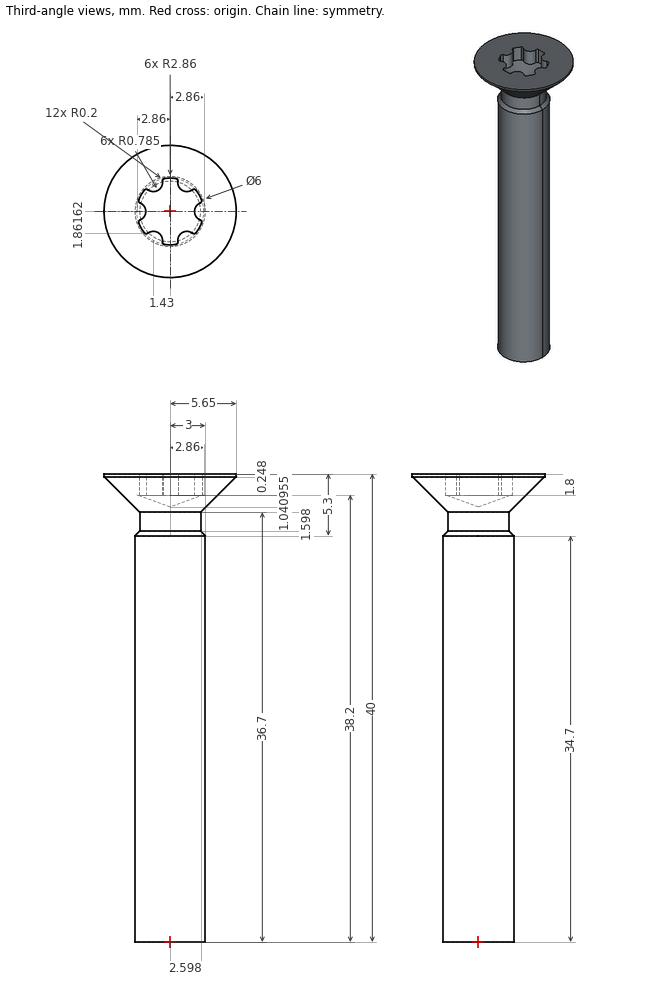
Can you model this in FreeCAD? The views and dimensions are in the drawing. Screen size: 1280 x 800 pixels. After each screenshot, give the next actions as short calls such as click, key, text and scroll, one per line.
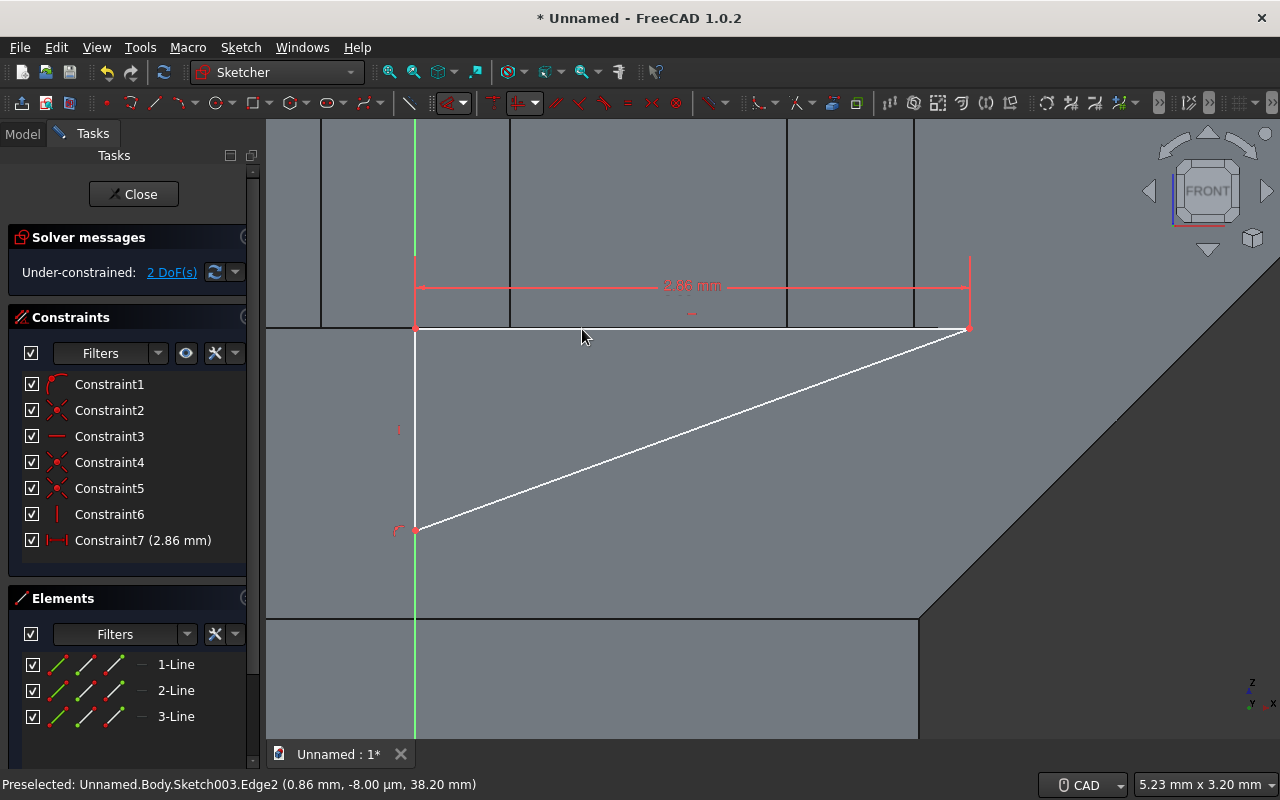
click(415, 329)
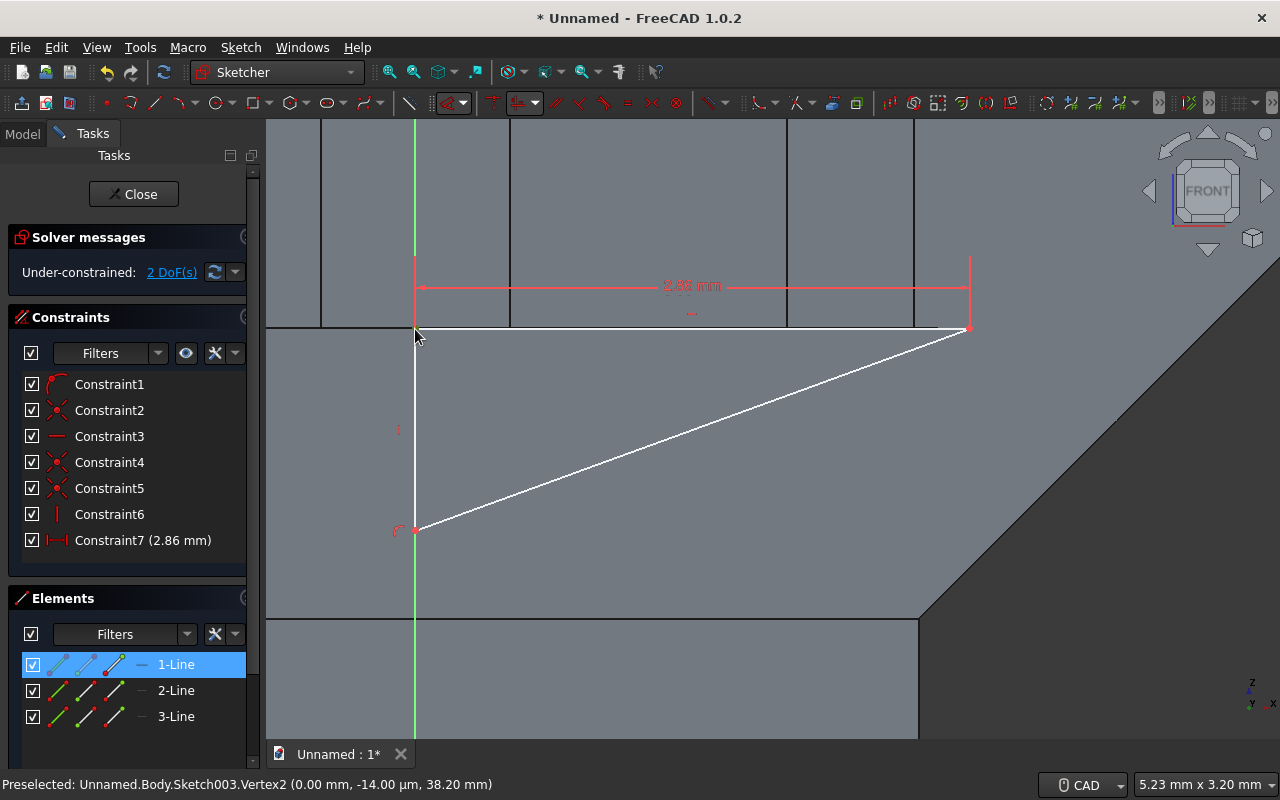
key(i)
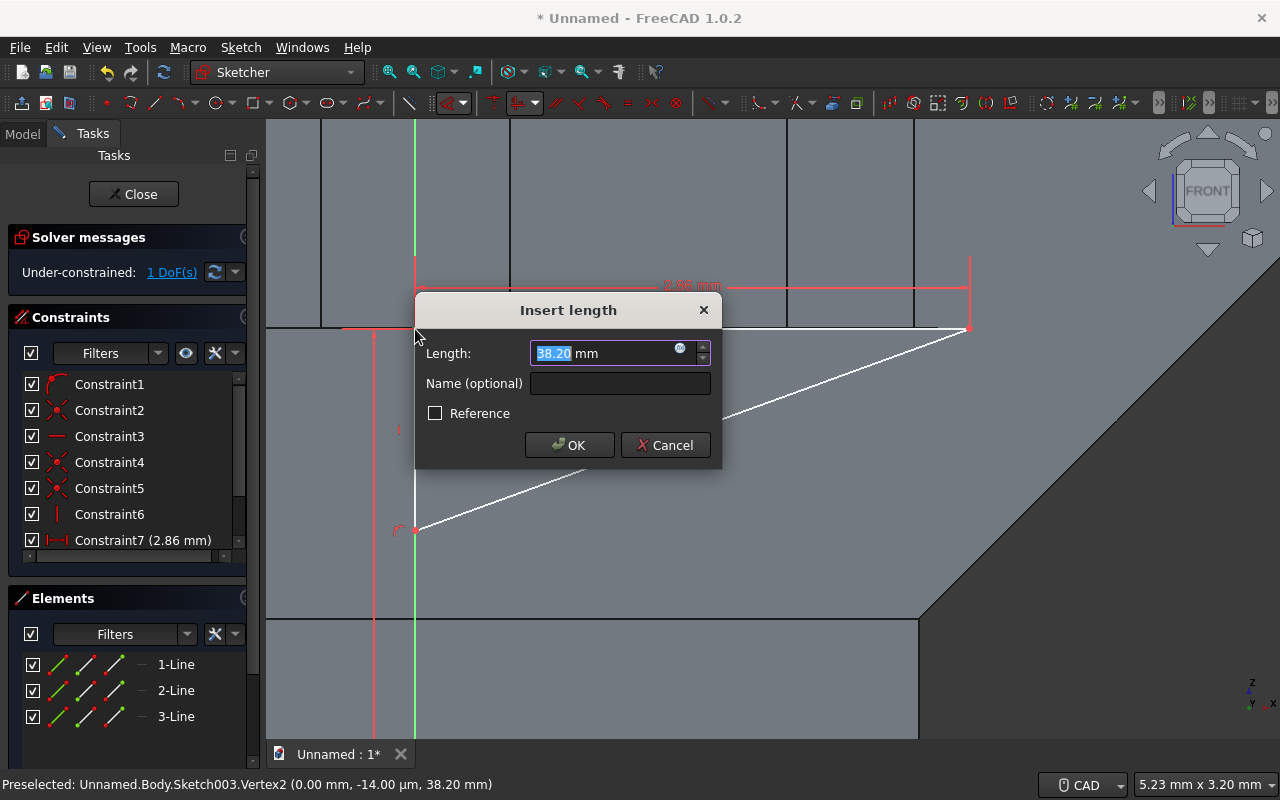
text(38.2)
key(Return)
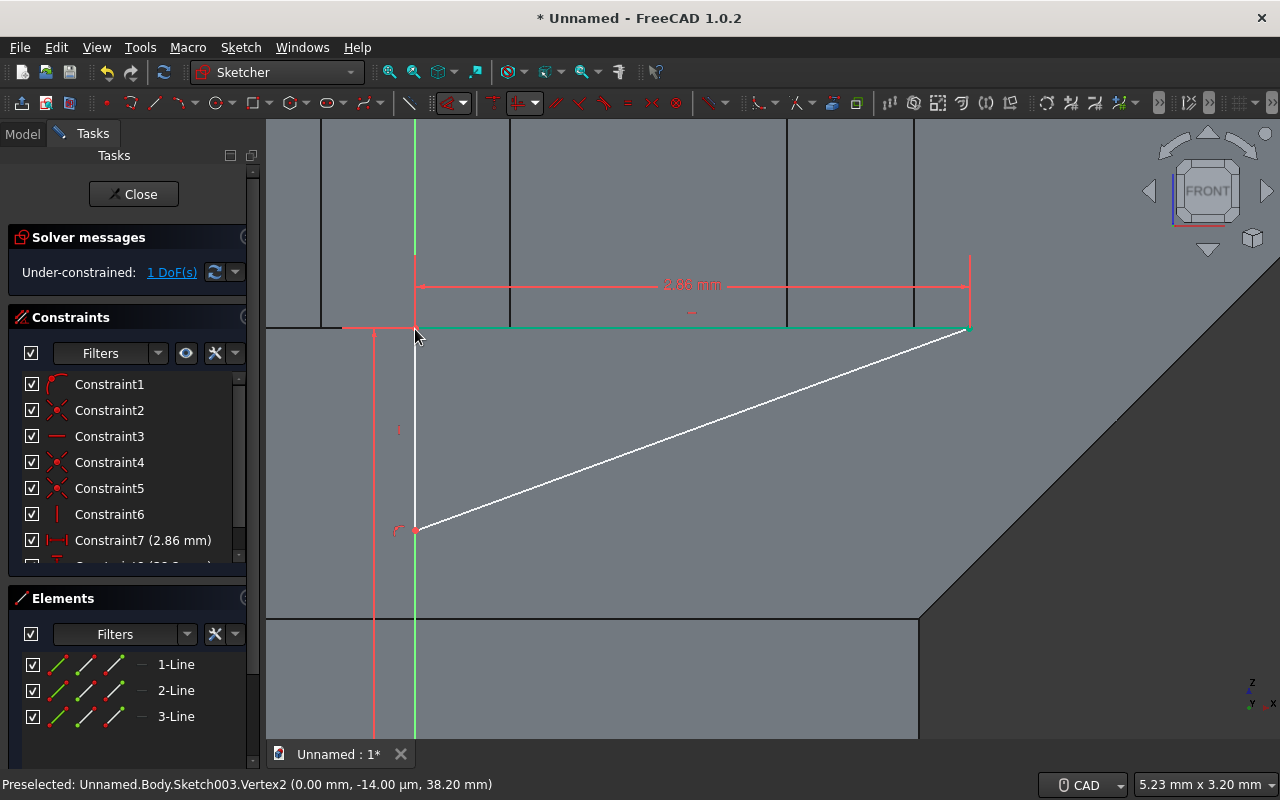
click(415, 470)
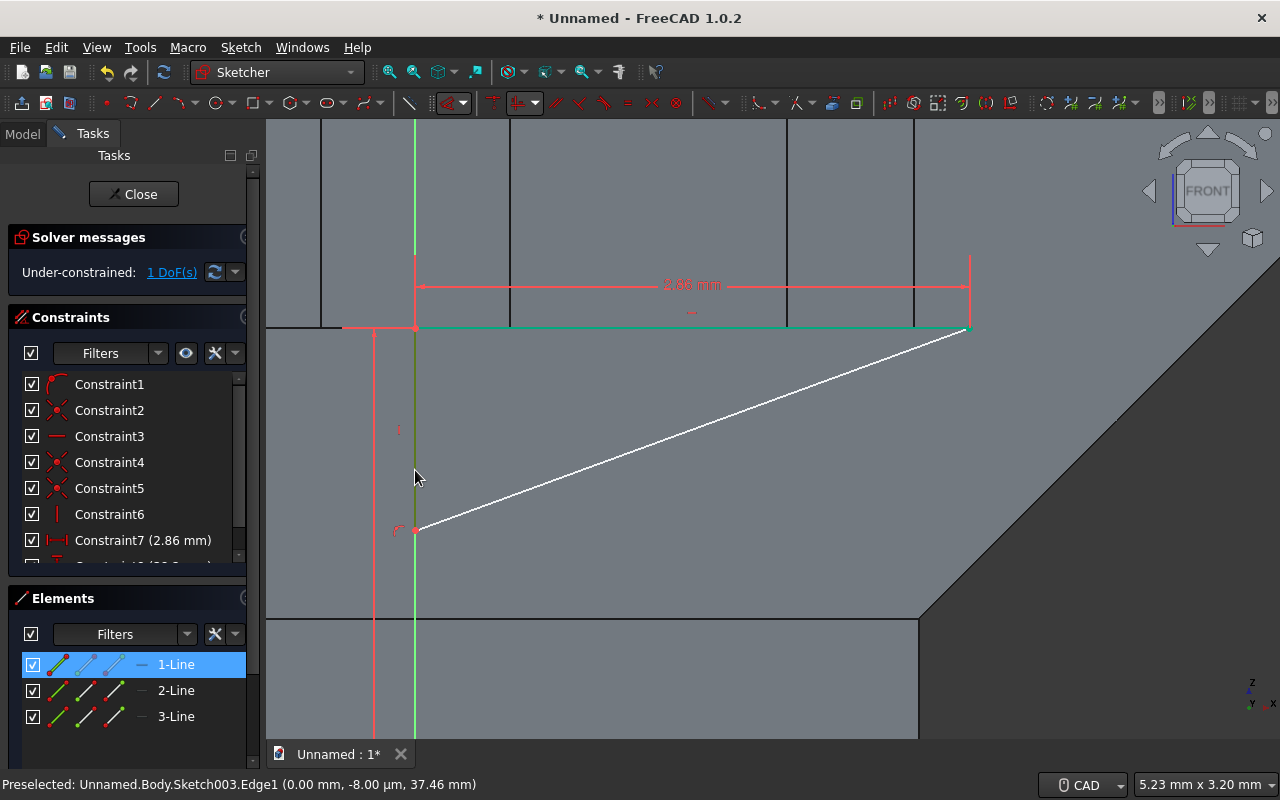
key(i)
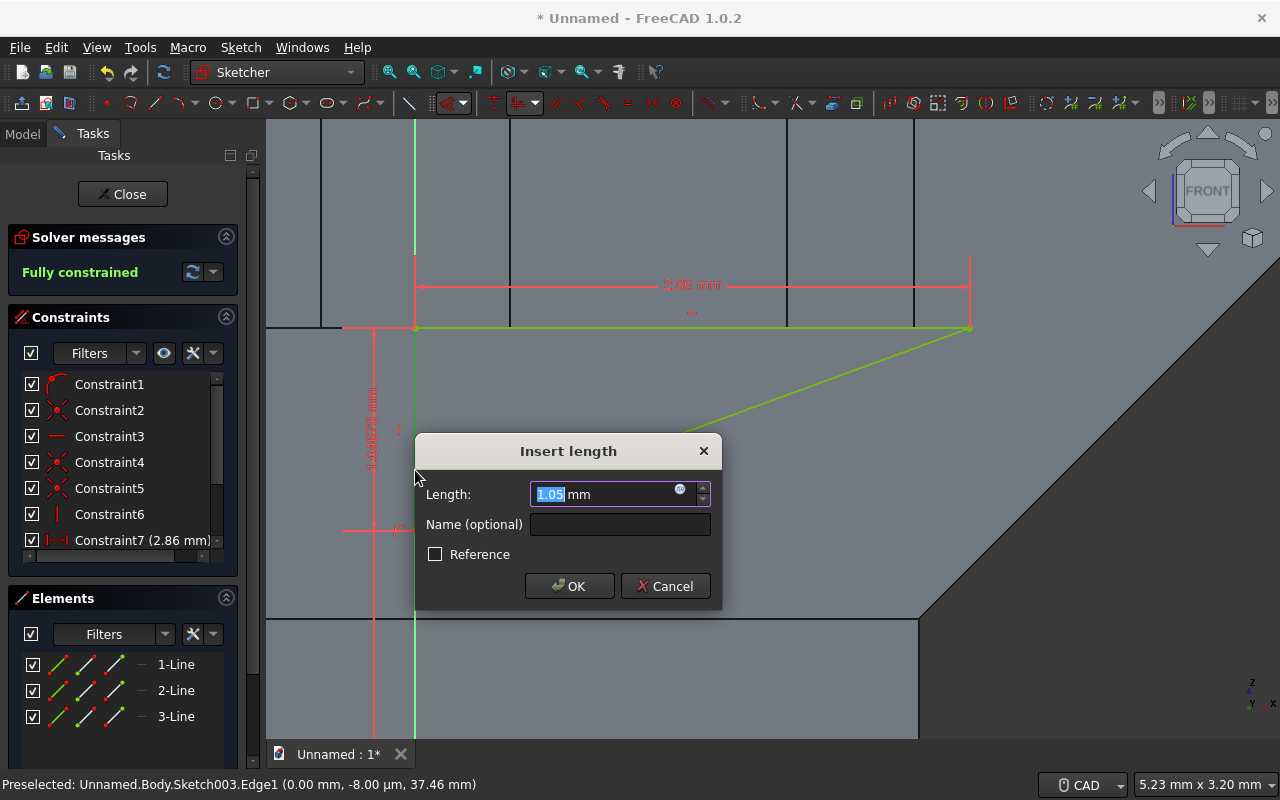
text(1.040955)
key(Return)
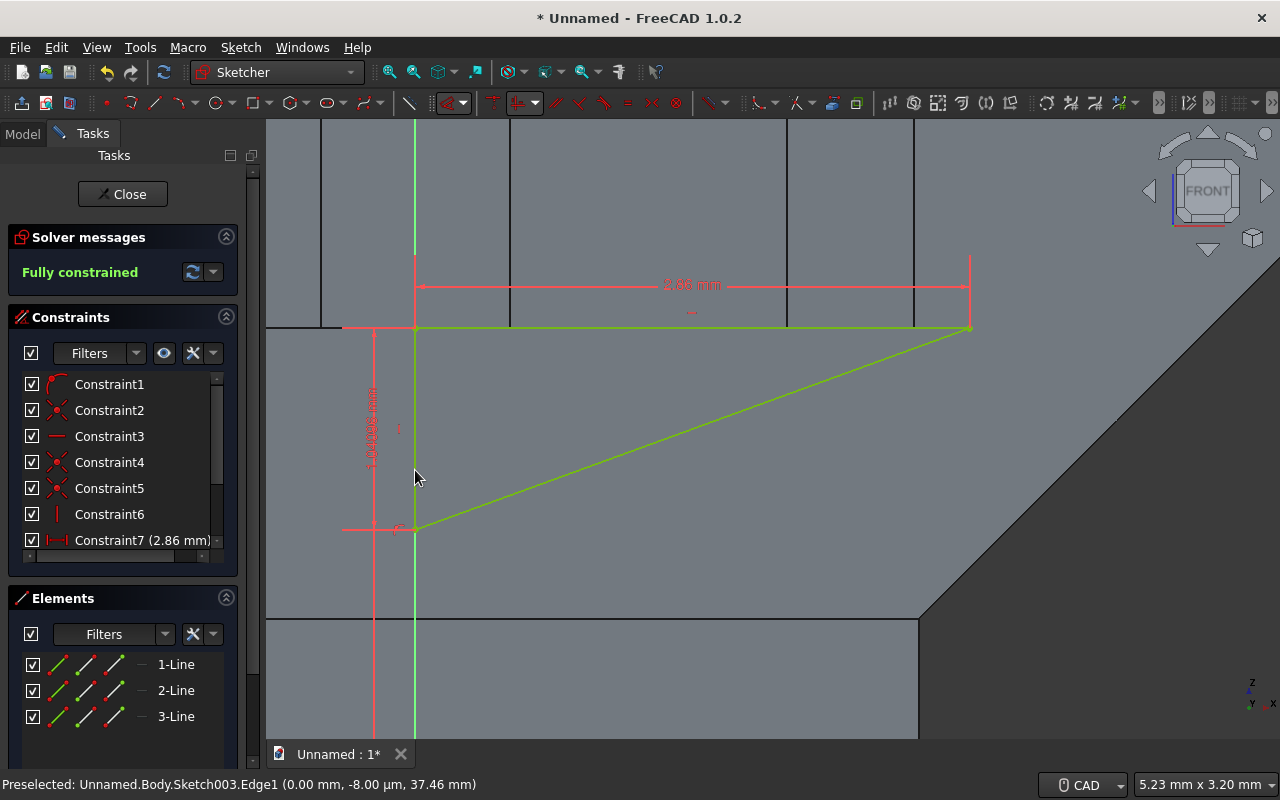
click(123, 194)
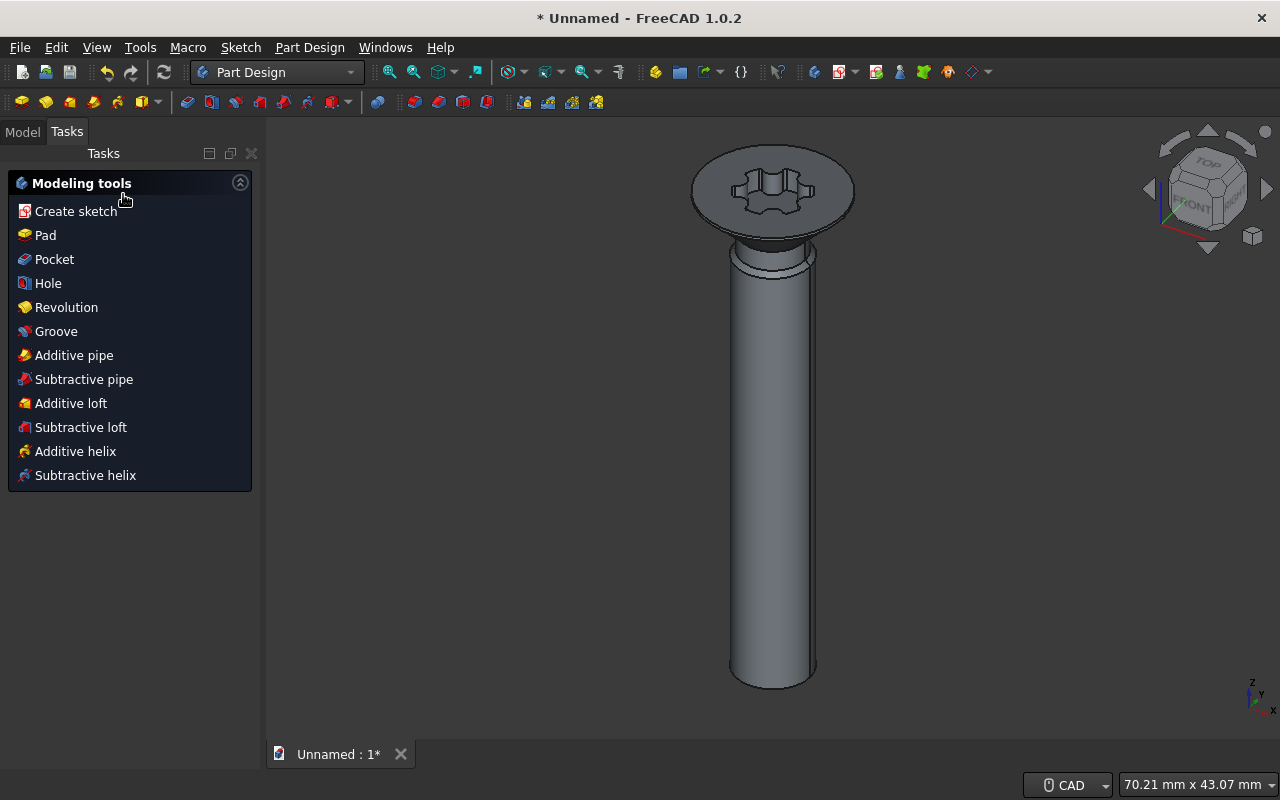
click(236, 102)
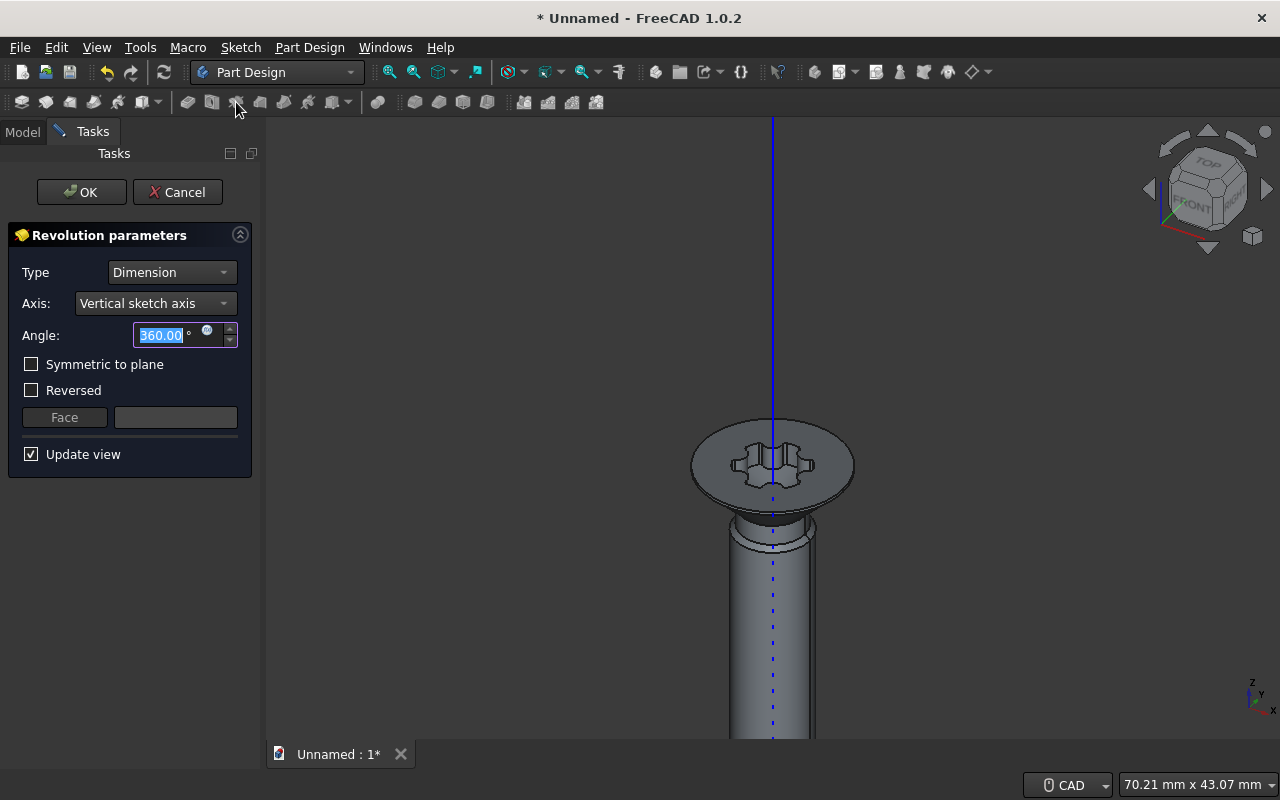
click(82, 192)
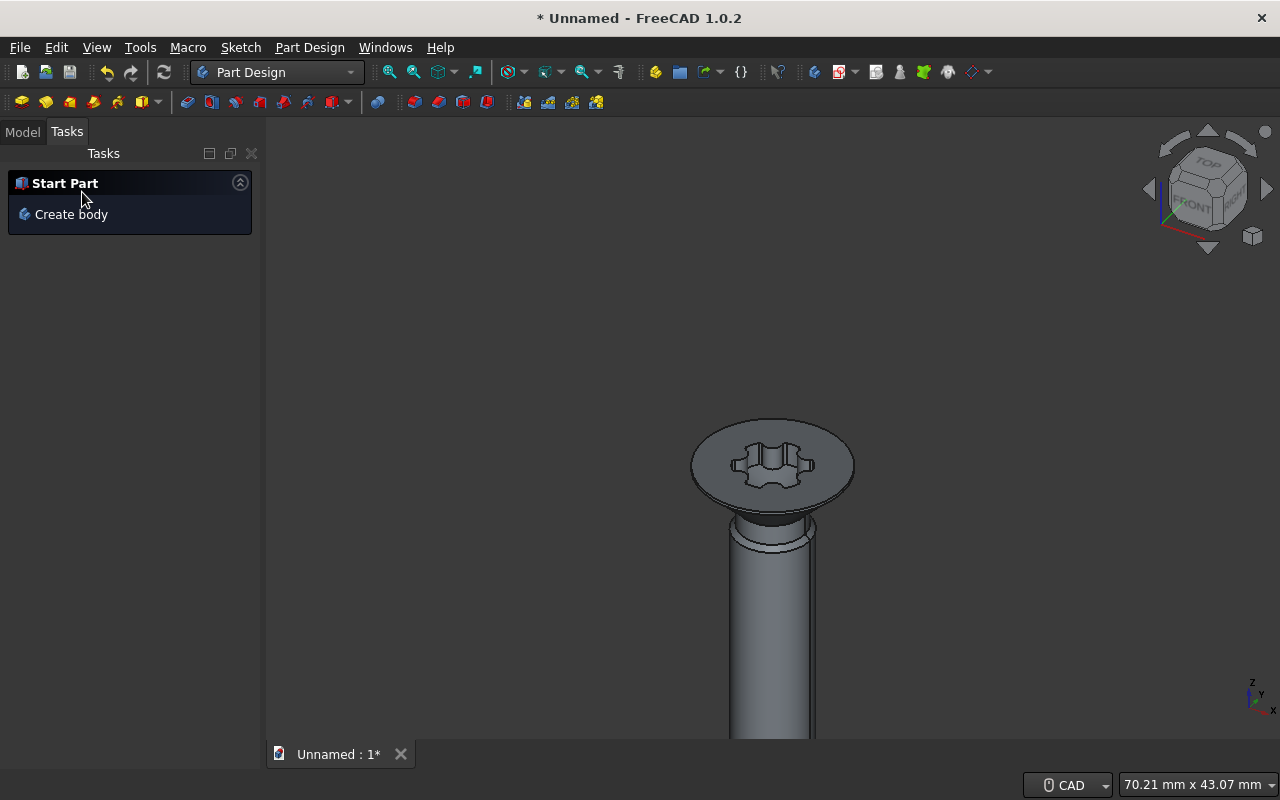
key(0)